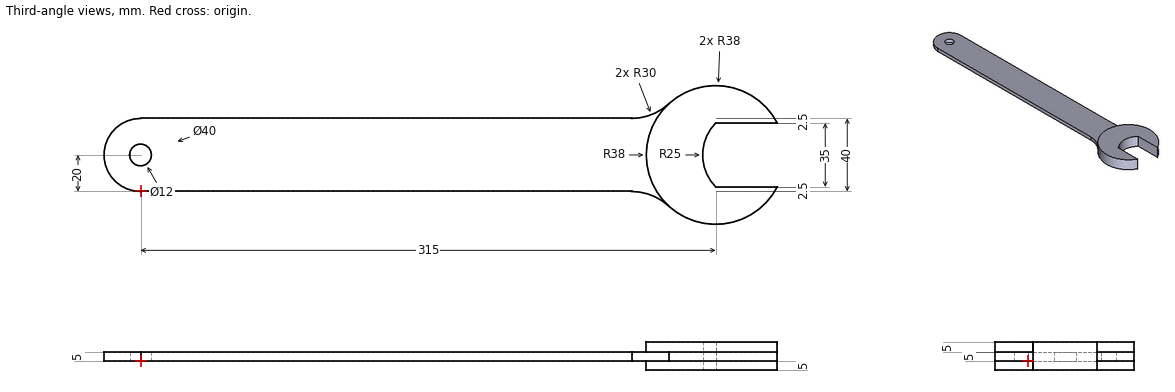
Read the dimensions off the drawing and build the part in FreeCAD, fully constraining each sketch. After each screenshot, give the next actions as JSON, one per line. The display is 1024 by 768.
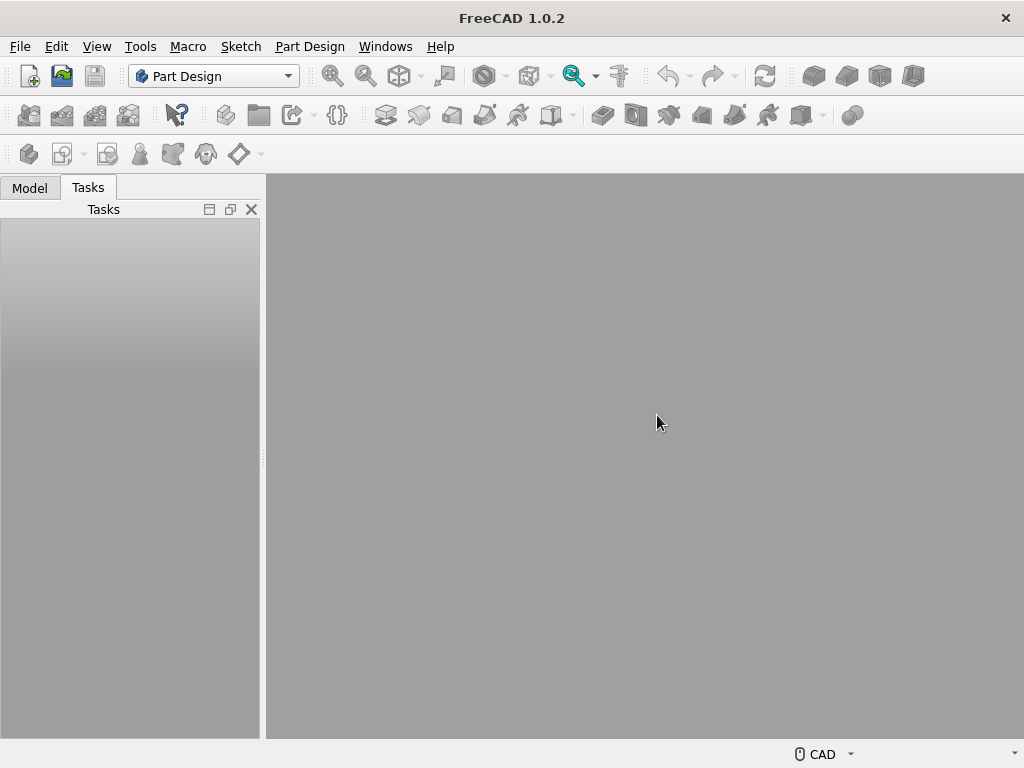
{"action": "left_click", "coordinate": [29, 76]}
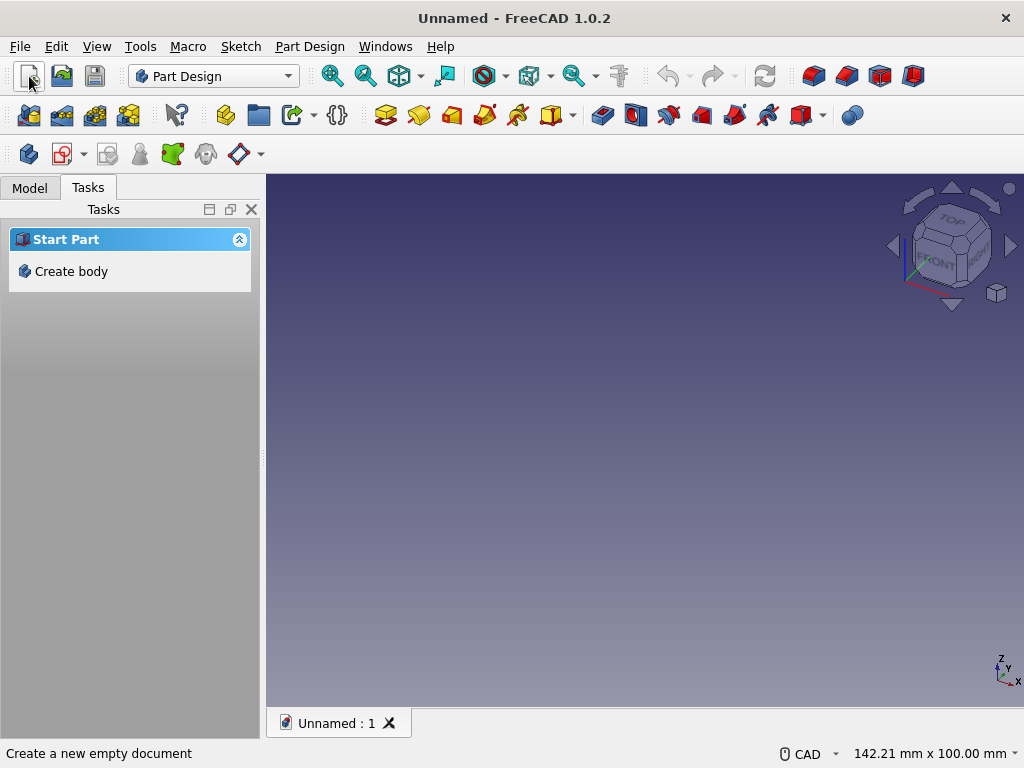
{"action": "left_click", "coordinate": [62, 154]}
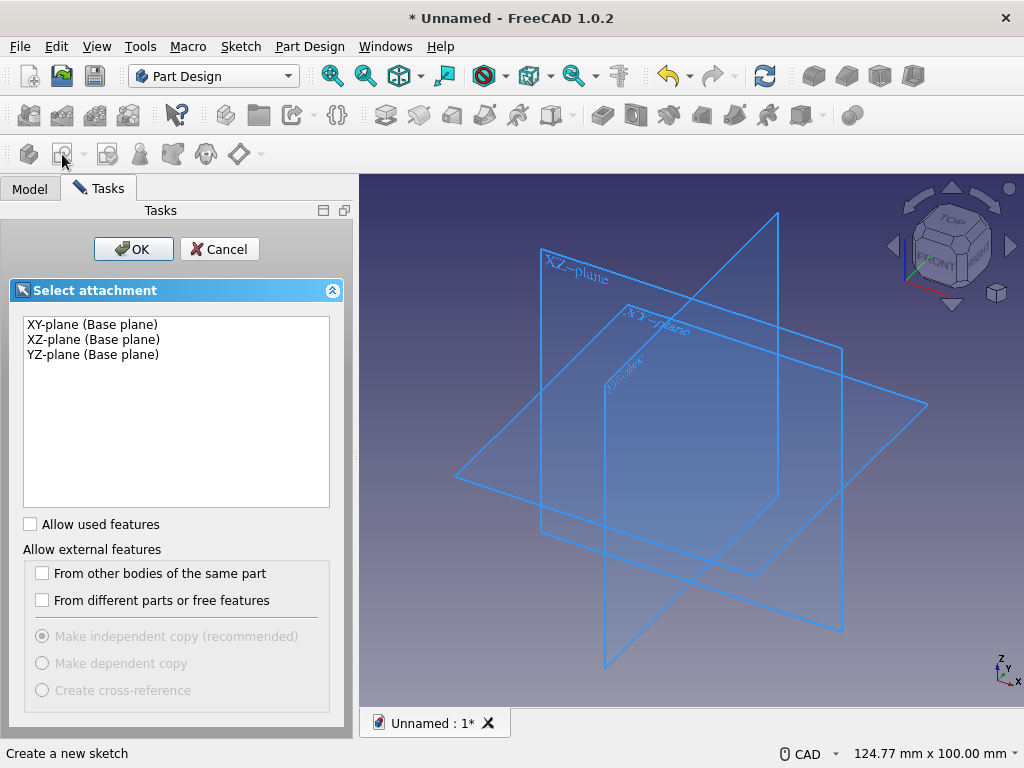
{"action": "left_click", "coordinate": [84, 324]}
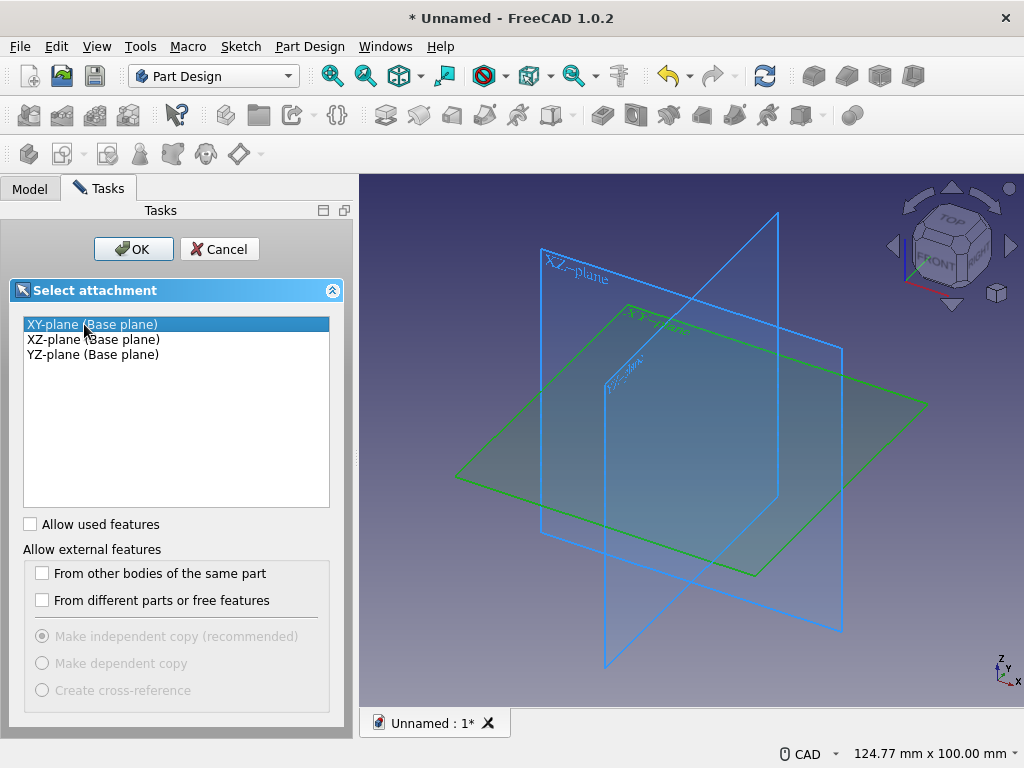
{"action": "left_click", "coordinate": [134, 249]}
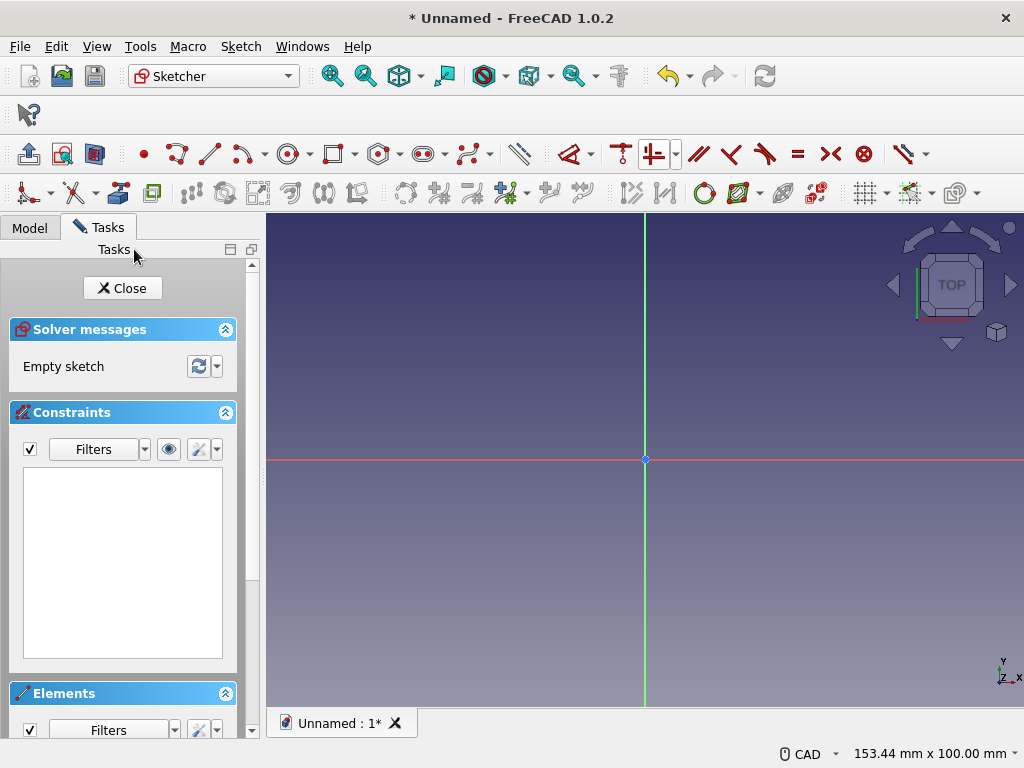
{"action": "scroll", "coordinate": [299, 492], "scroll_direction": "down", "scroll_amount": 7}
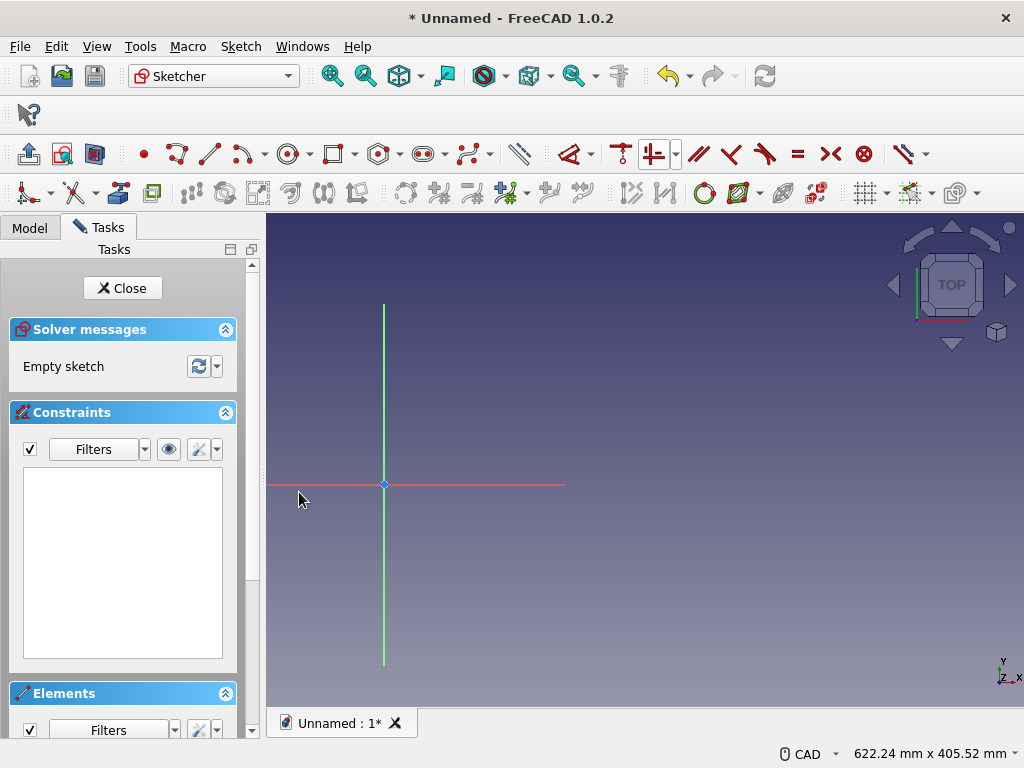
{"action": "left_click", "coordinate": [332, 154]}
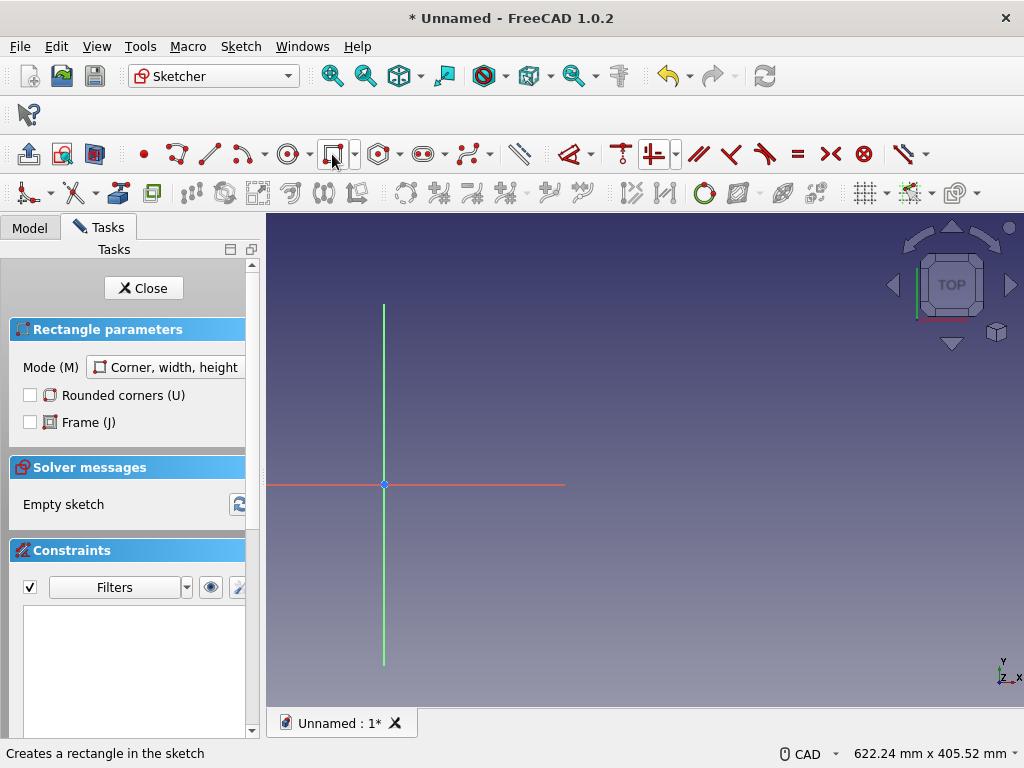
{"action": "left_click", "coordinate": [384, 485]}
{"action": "mouse_move", "coordinate": [768, 436]}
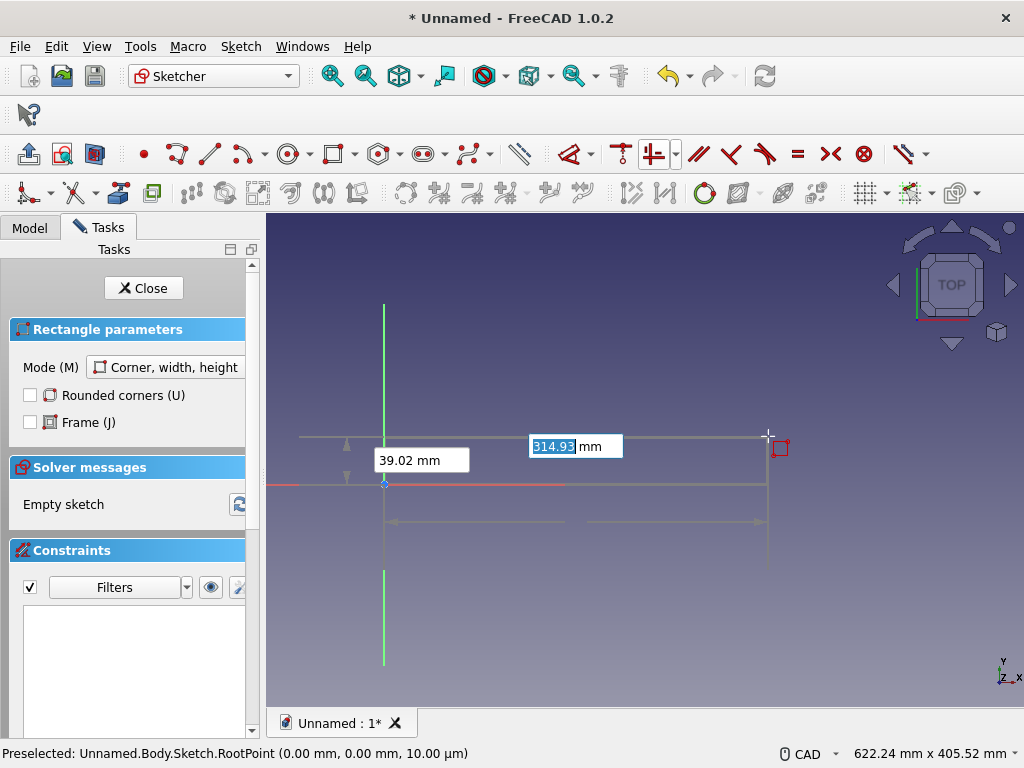
{"action": "type", "text": "315"}
{"action": "key", "text": "Tab"}
{"action": "type", "text": "40"}
{"action": "key", "text": "Return"}
{"action": "key", "text": "Escape"}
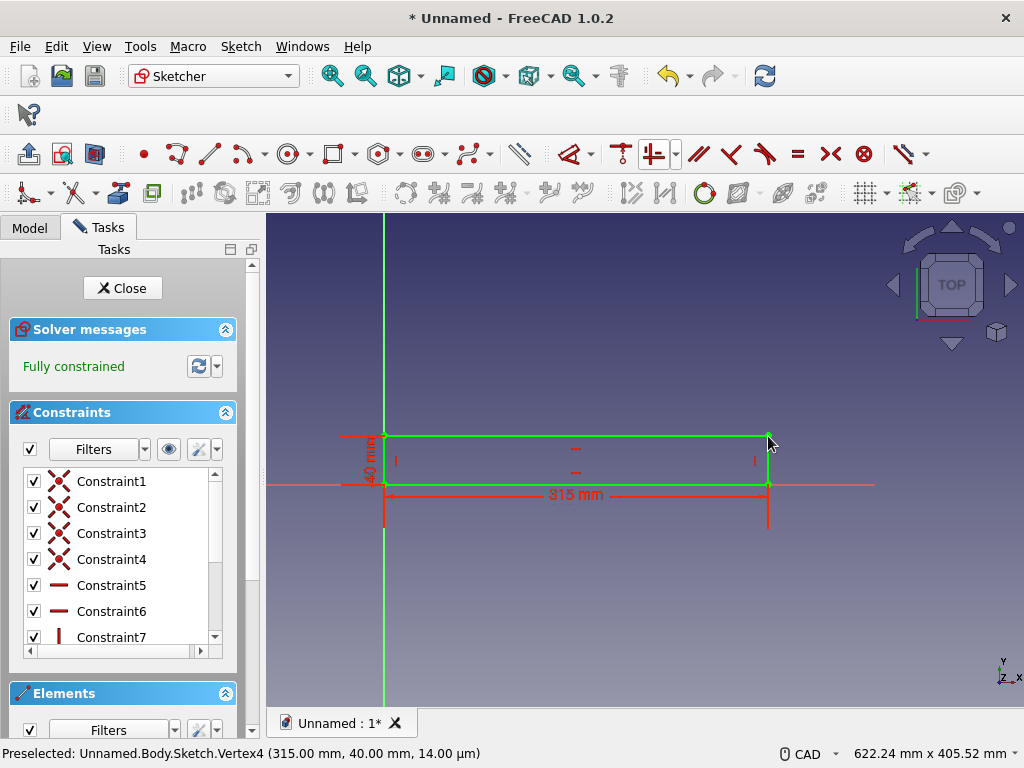
{"action": "left_click", "coordinate": [123, 288]}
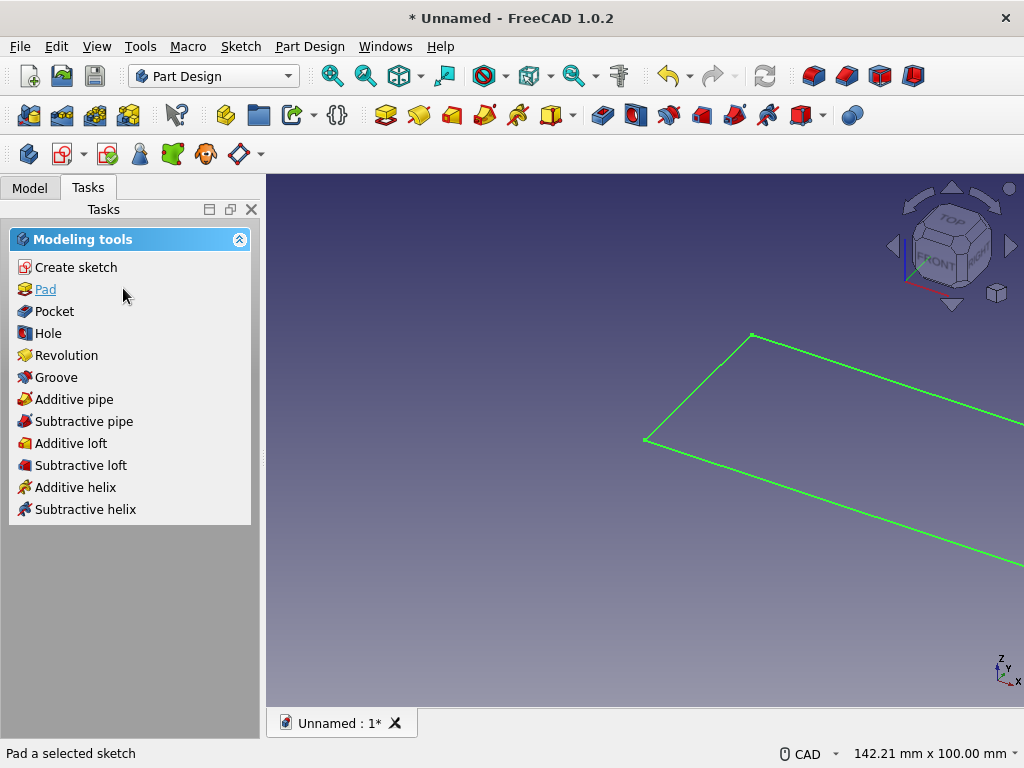
{"action": "left_click", "coordinate": [386, 116]}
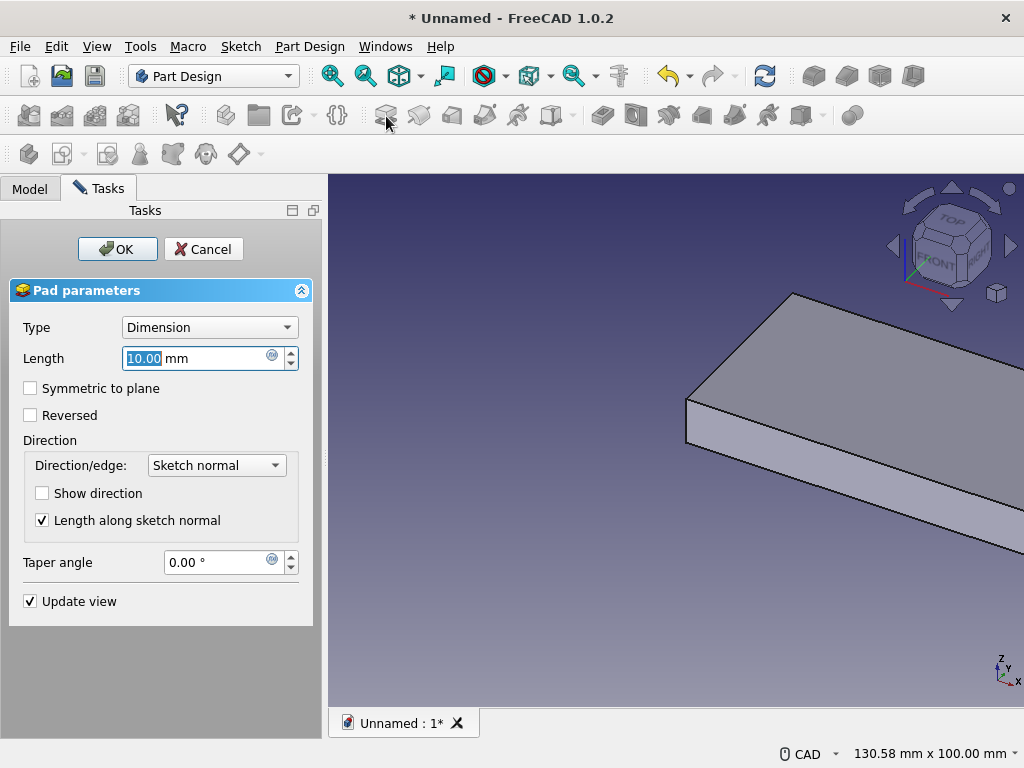
{"action": "type", "text": "5"}
{"action": "key", "text": "Tab"}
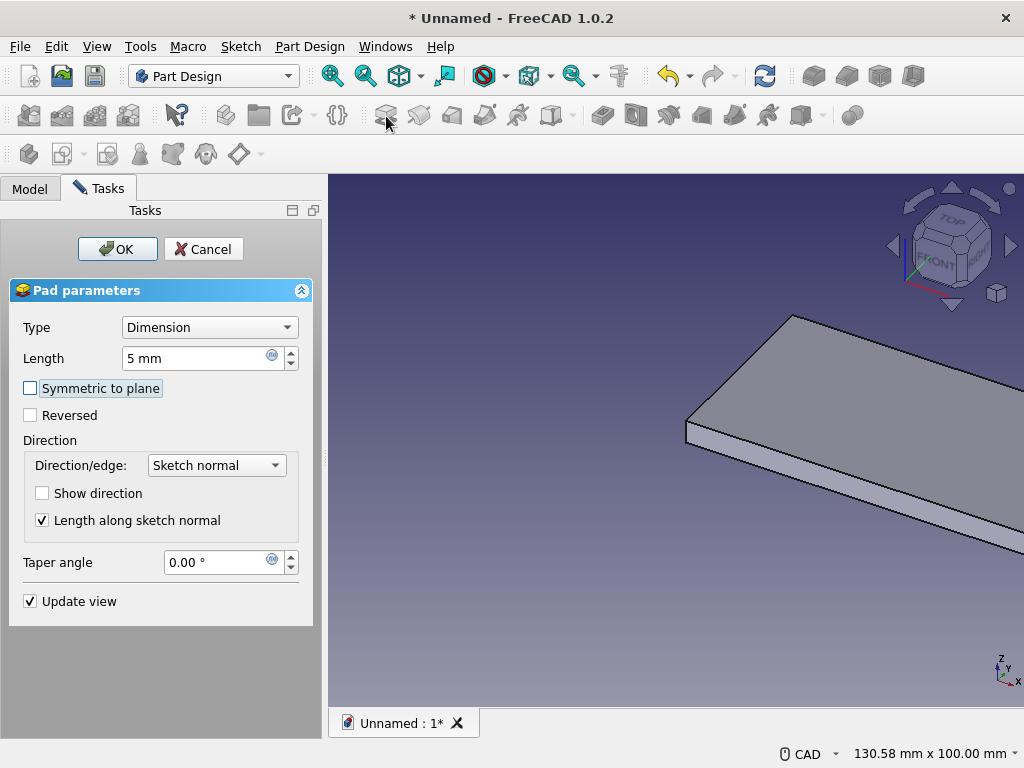
{"action": "left_click", "coordinate": [118, 249]}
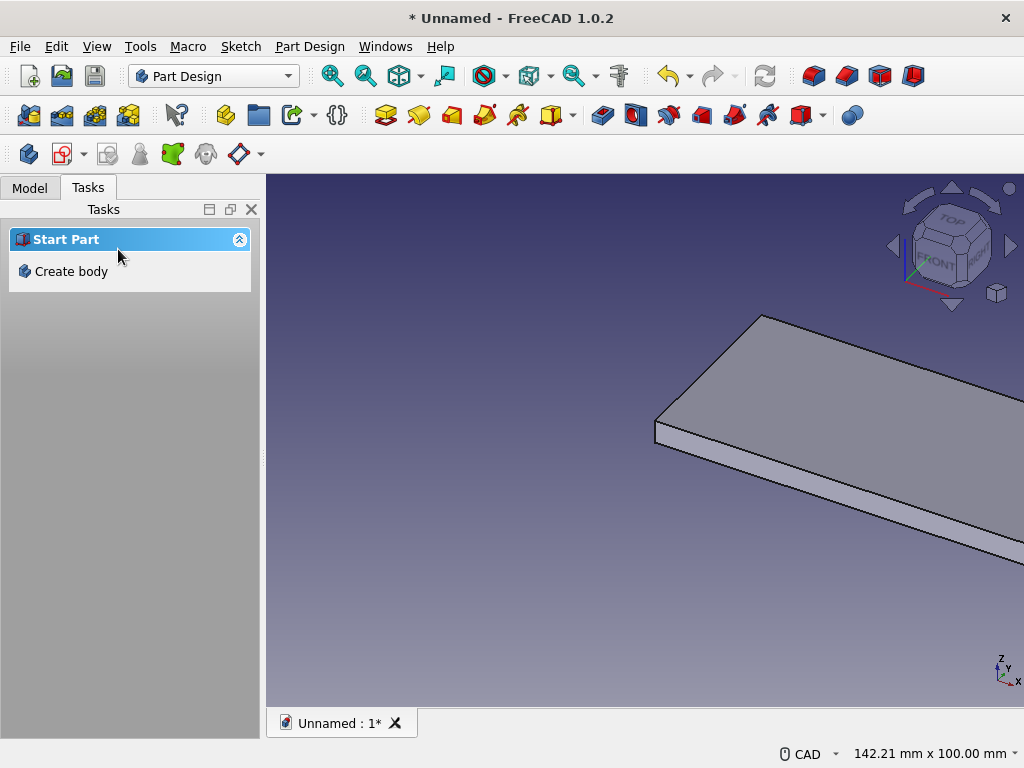
{"action": "left_click", "coordinate": [333, 76]}